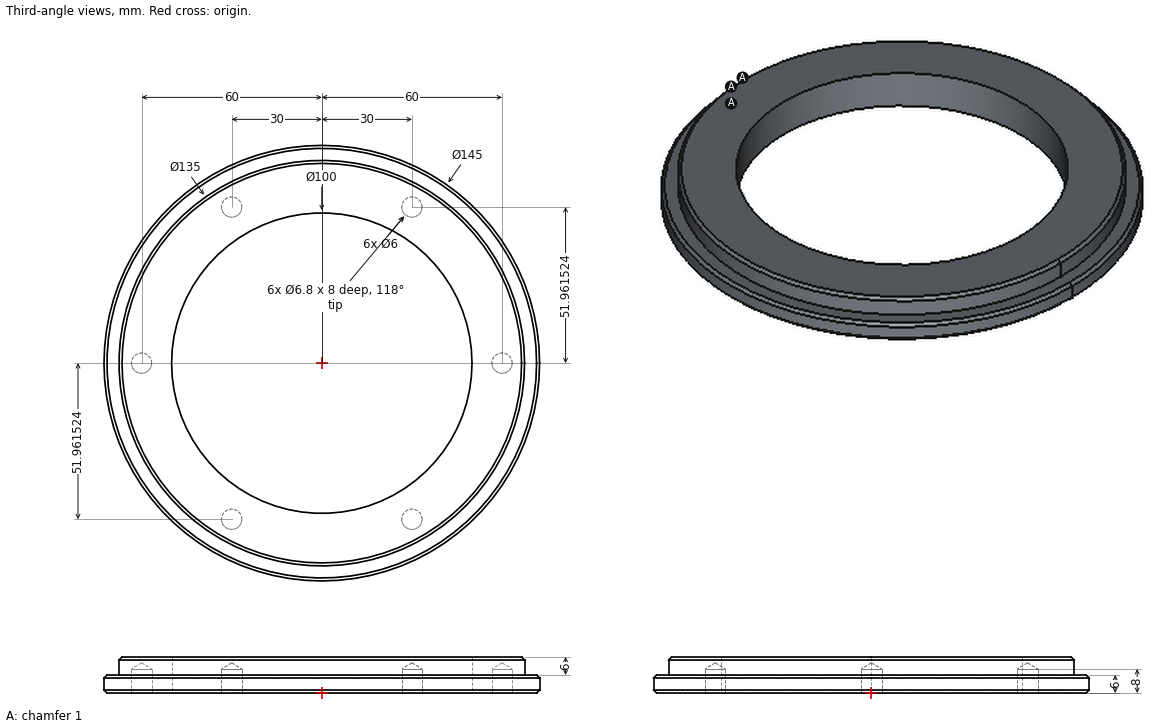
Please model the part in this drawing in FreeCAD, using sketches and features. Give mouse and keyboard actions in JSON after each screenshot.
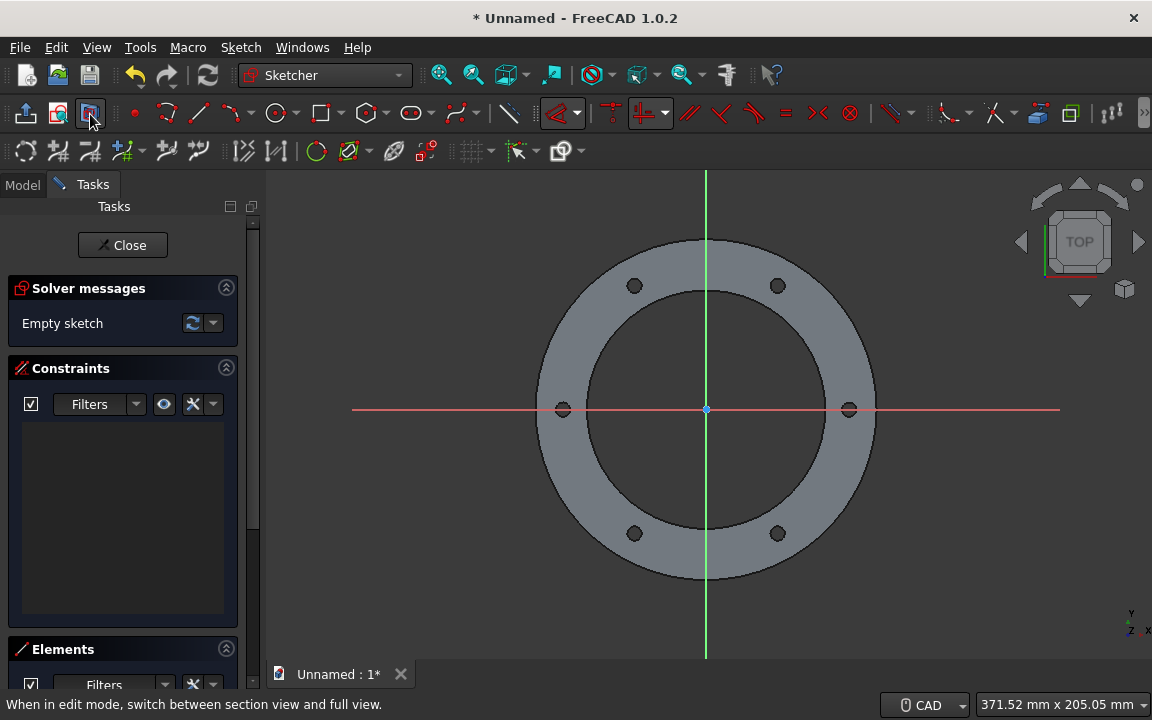
{"action": "left_click", "coordinate": [276, 114]}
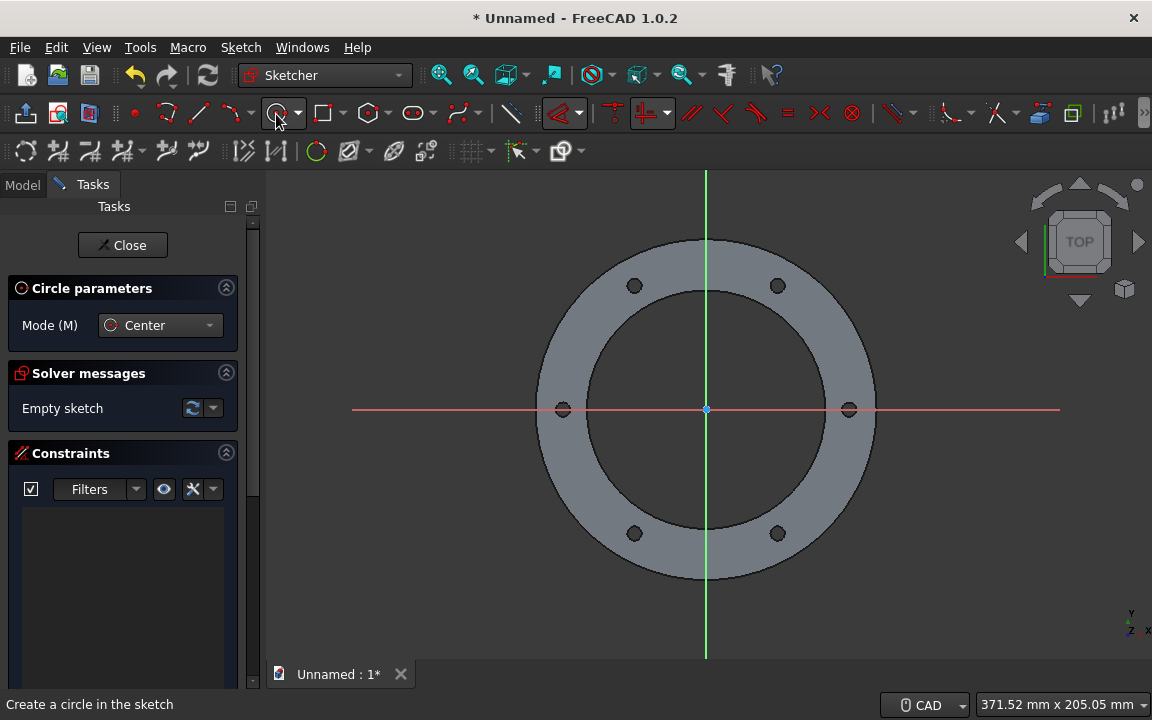
{"action": "scroll", "coordinate": [778, 286], "scroll_direction": "up", "scroll_amount": 6}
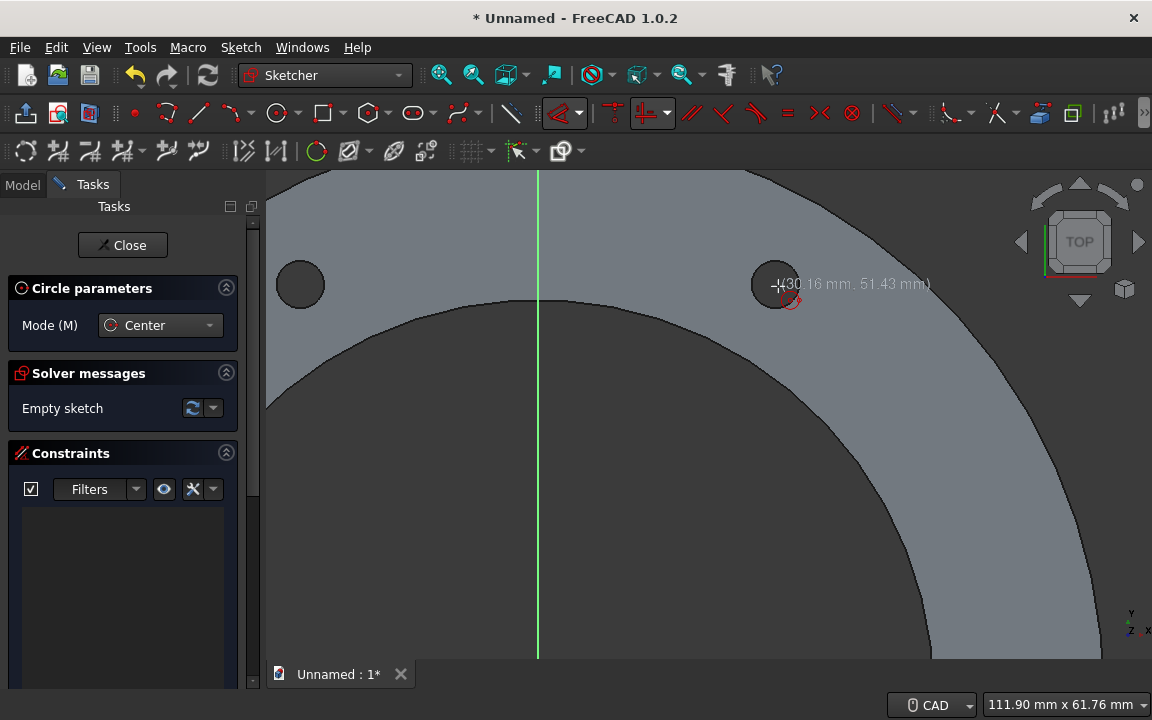
{"action": "left_click", "coordinate": [775, 285]}
{"action": "mouse_move", "coordinate": [794, 266]}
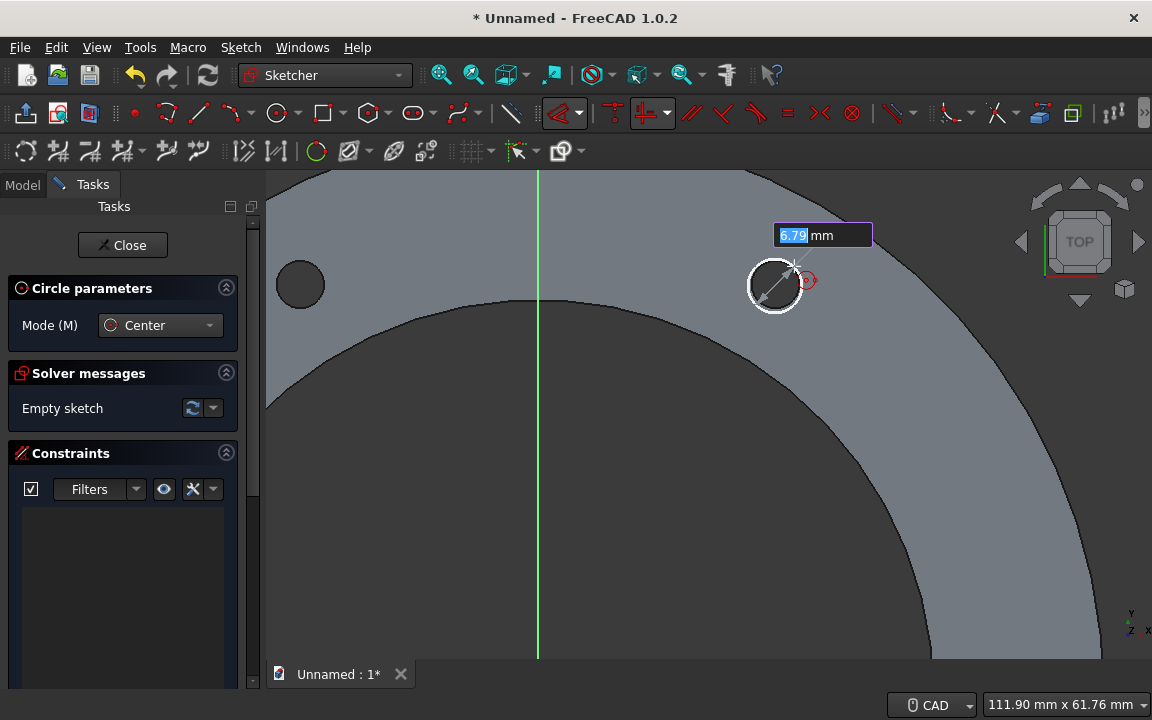
{"action": "type", "text": "6.8"}
{"action": "key", "text": "Return"}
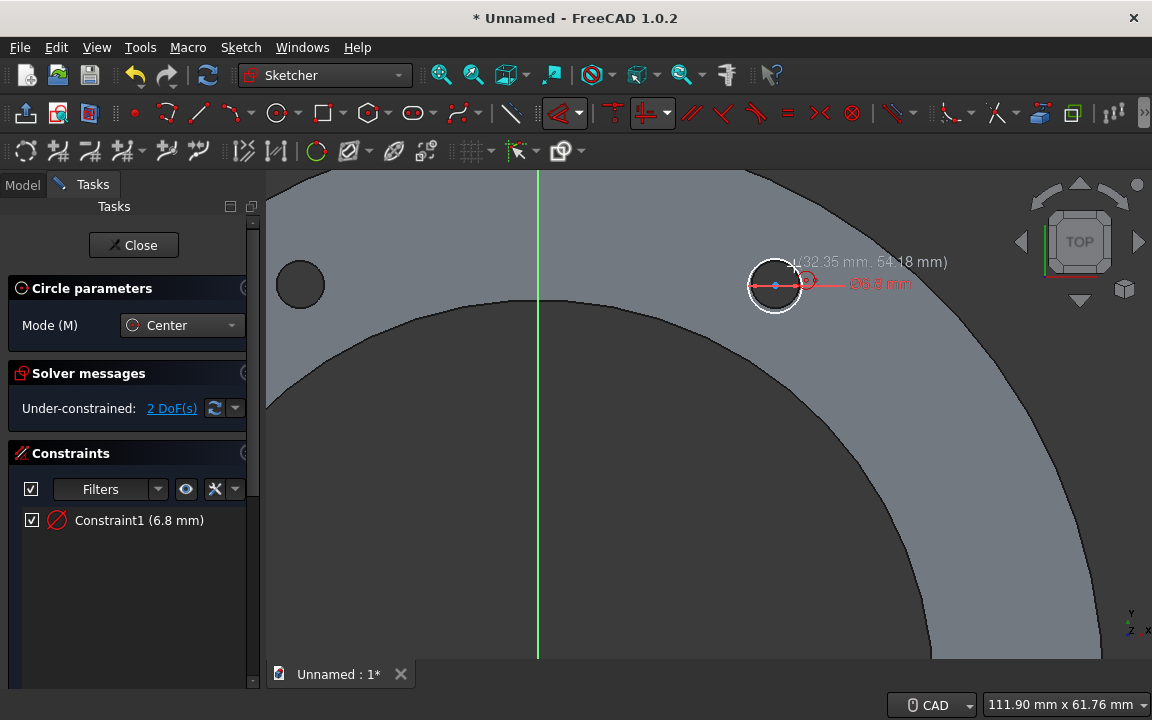
{"action": "left_click", "coordinate": [300, 285]}
{"action": "mouse_move", "coordinate": [319, 266]}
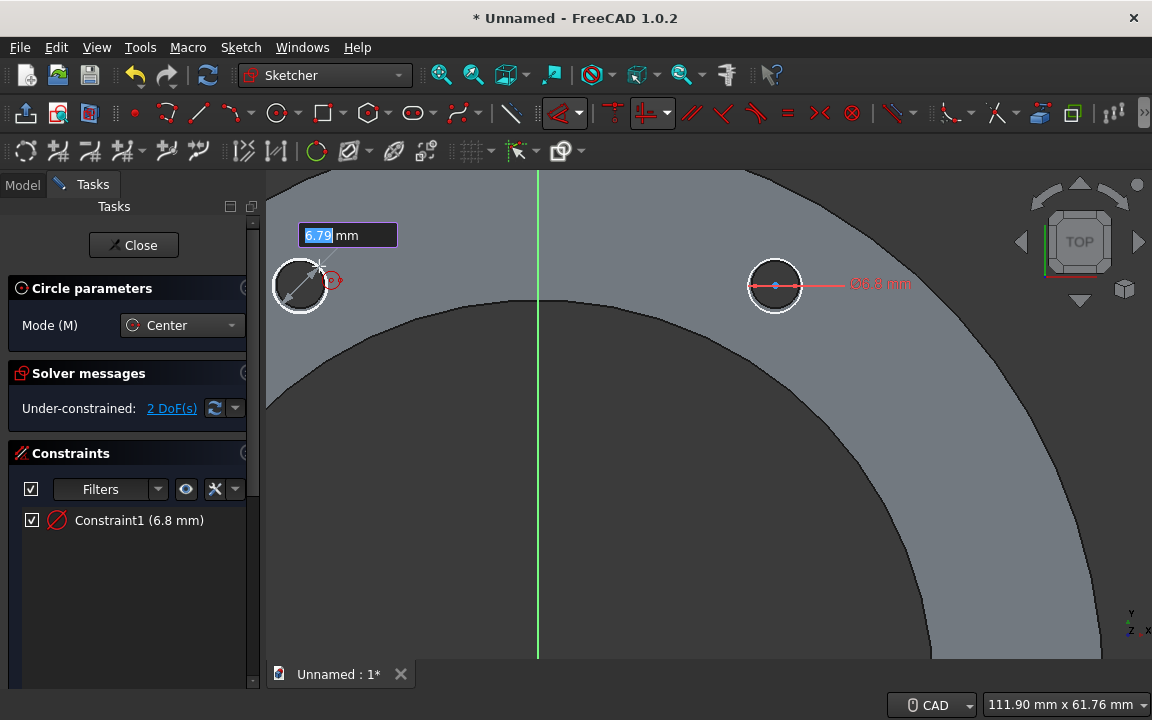
{"action": "type", "text": "6.8"}
{"action": "key", "text": "Return"}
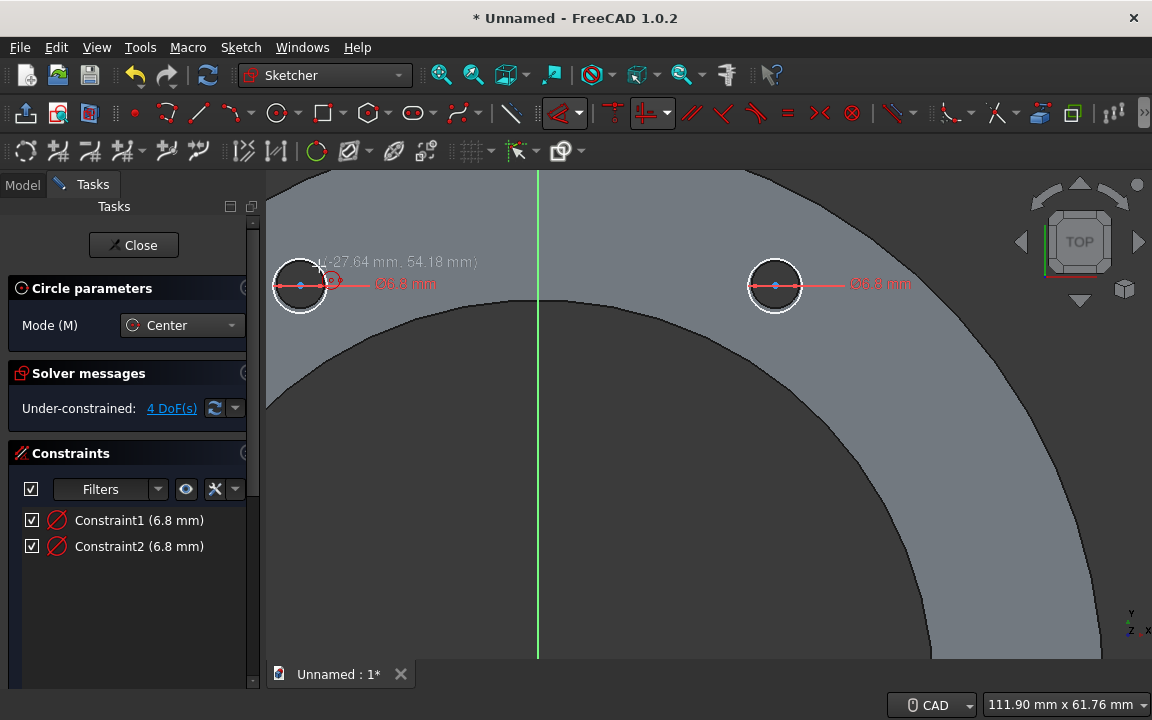
{"action": "scroll", "coordinate": [700, 251], "scroll_direction": "down", "scroll_amount": 5}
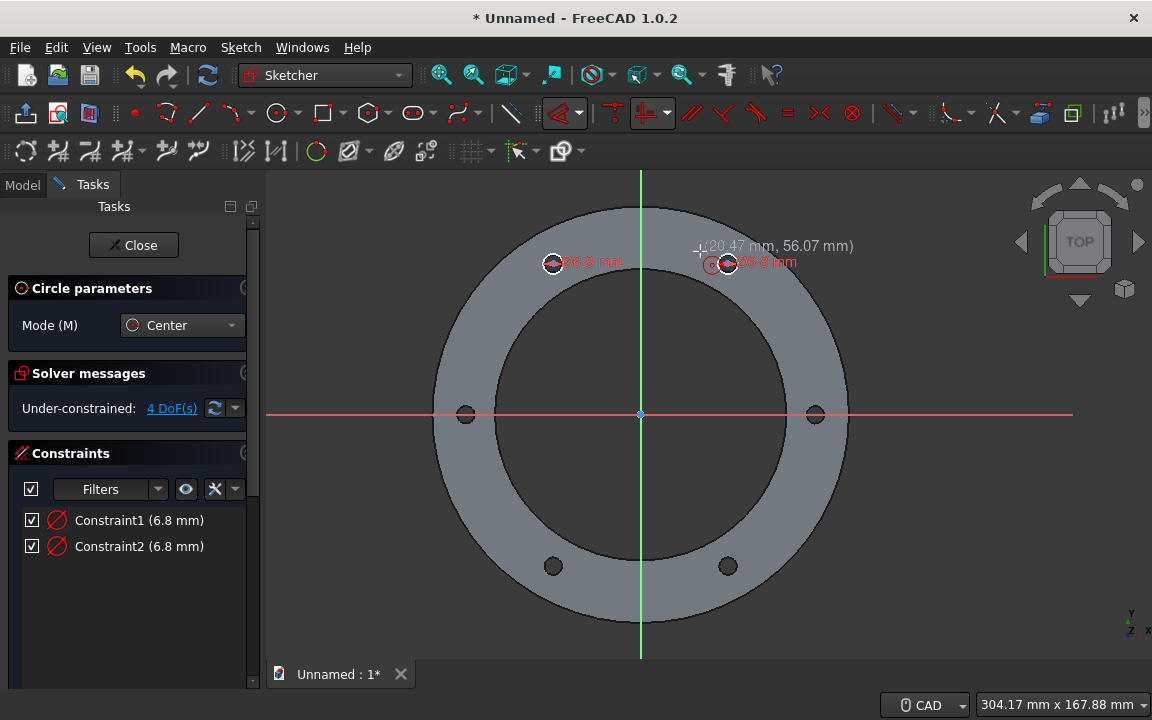
{"action": "scroll", "coordinate": [466, 415], "scroll_direction": "up", "scroll_amount": 5}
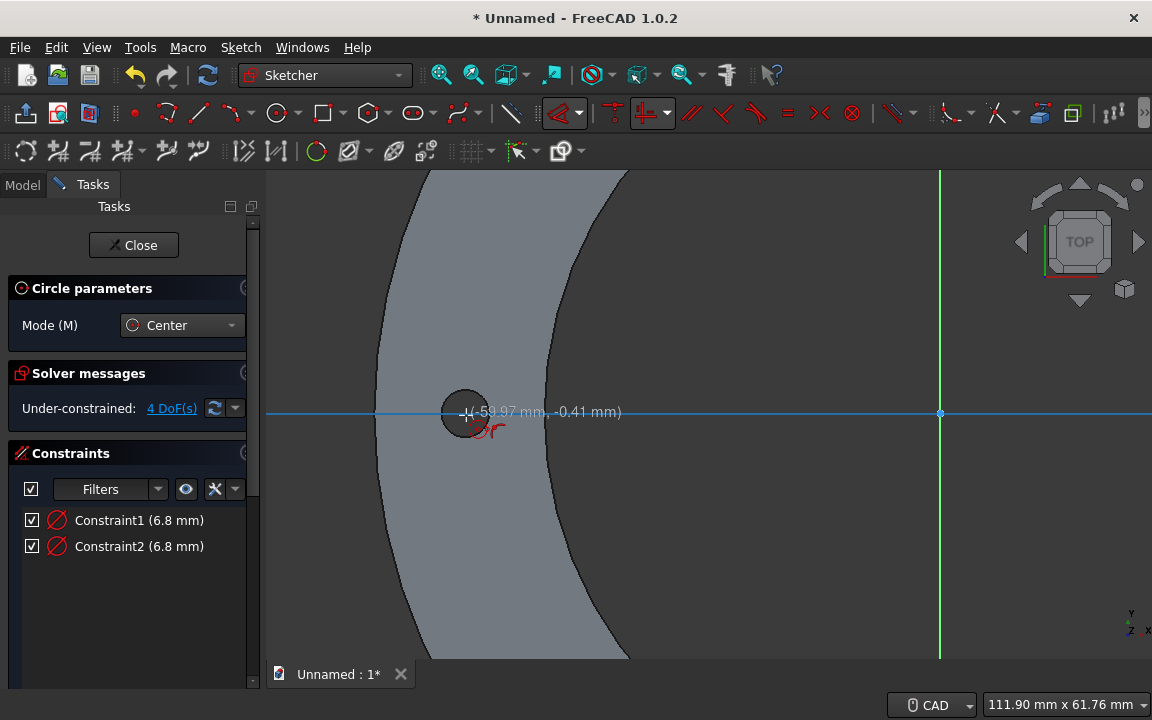
{"action": "left_click", "coordinate": [465, 414]}
{"action": "mouse_move", "coordinate": [484, 395]}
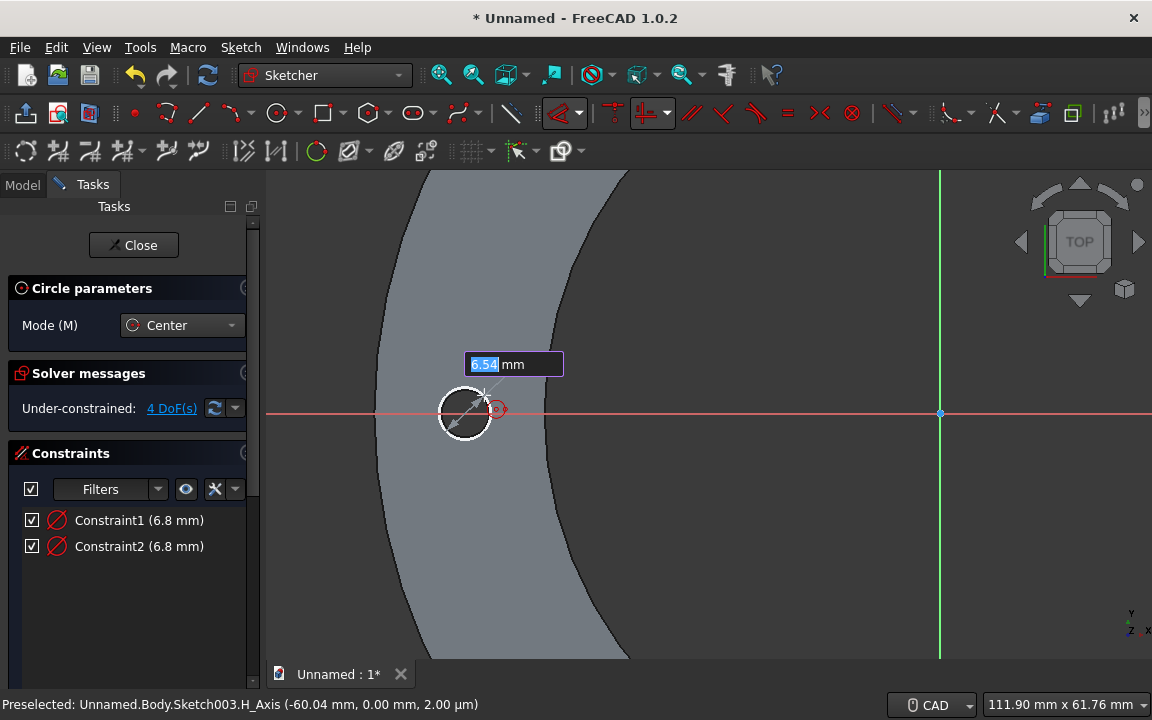
{"action": "type", "text": "6.8"}
{"action": "key", "text": "Return"}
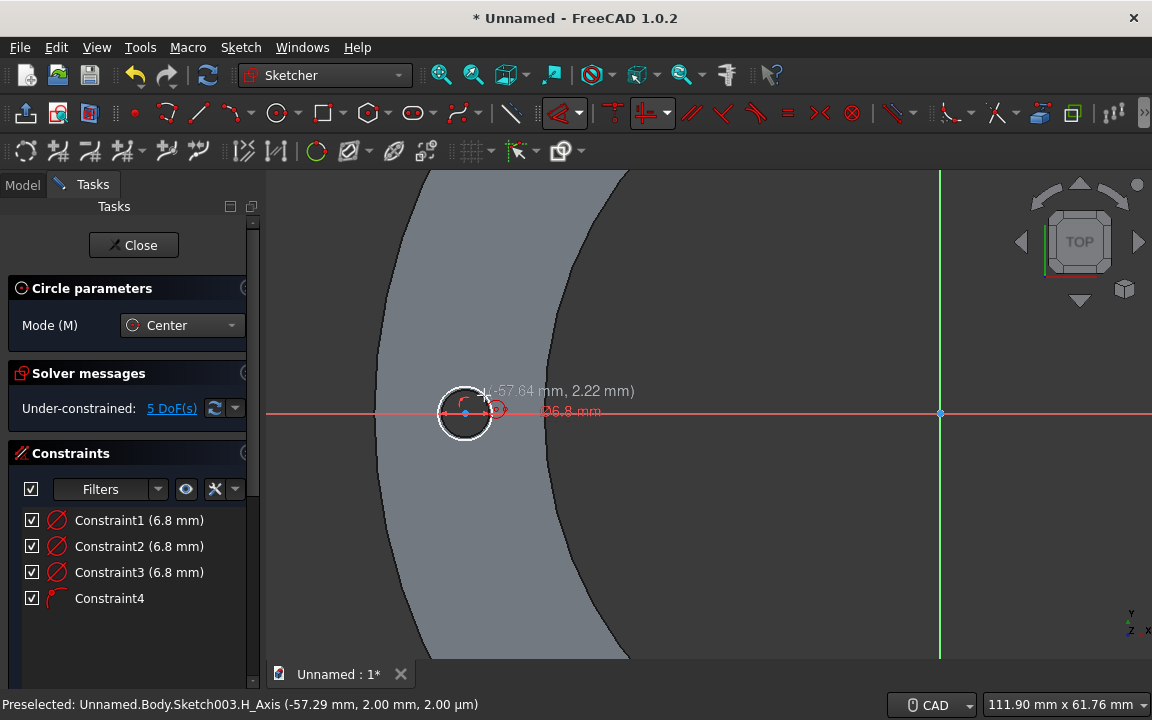
{"action": "scroll", "coordinate": [466, 415], "scroll_direction": "down", "scroll_amount": 5}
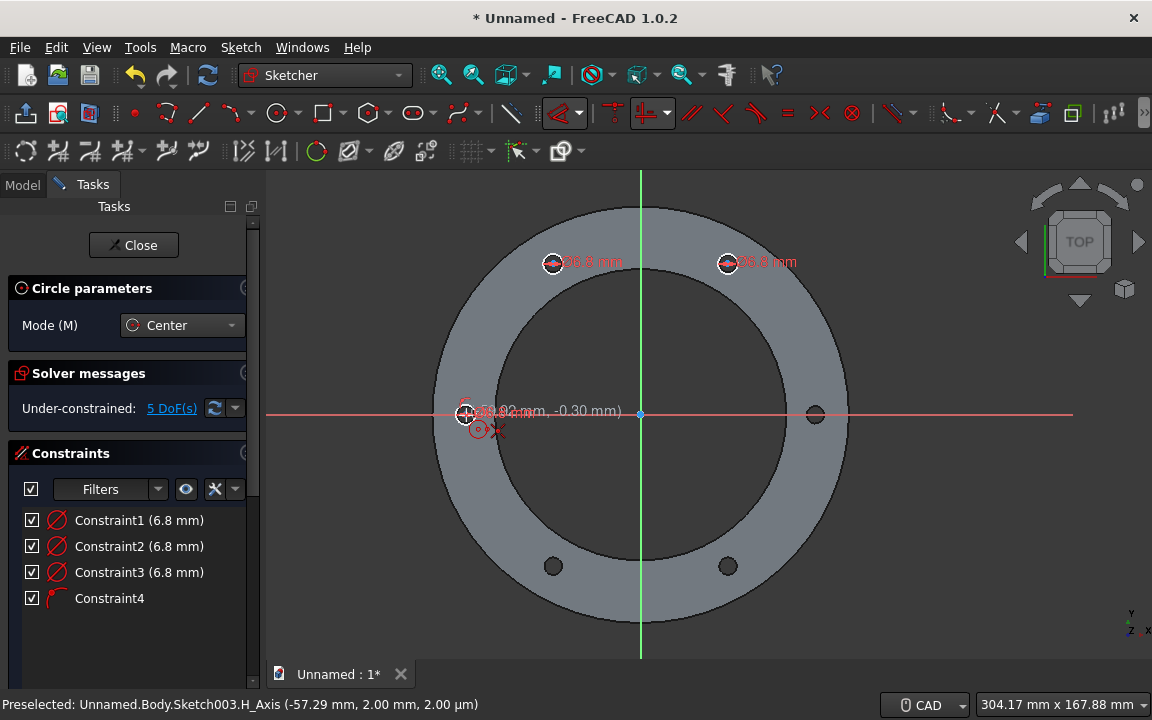
{"action": "scroll", "coordinate": [553, 566], "scroll_direction": "up", "scroll_amount": 5}